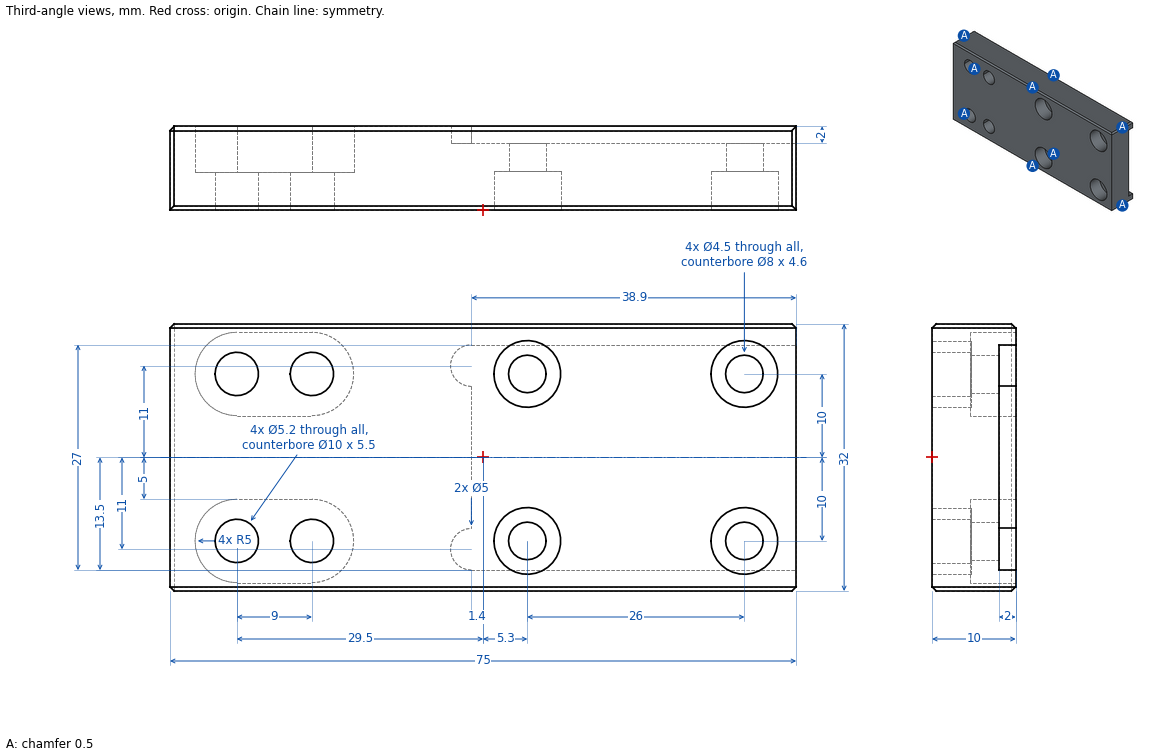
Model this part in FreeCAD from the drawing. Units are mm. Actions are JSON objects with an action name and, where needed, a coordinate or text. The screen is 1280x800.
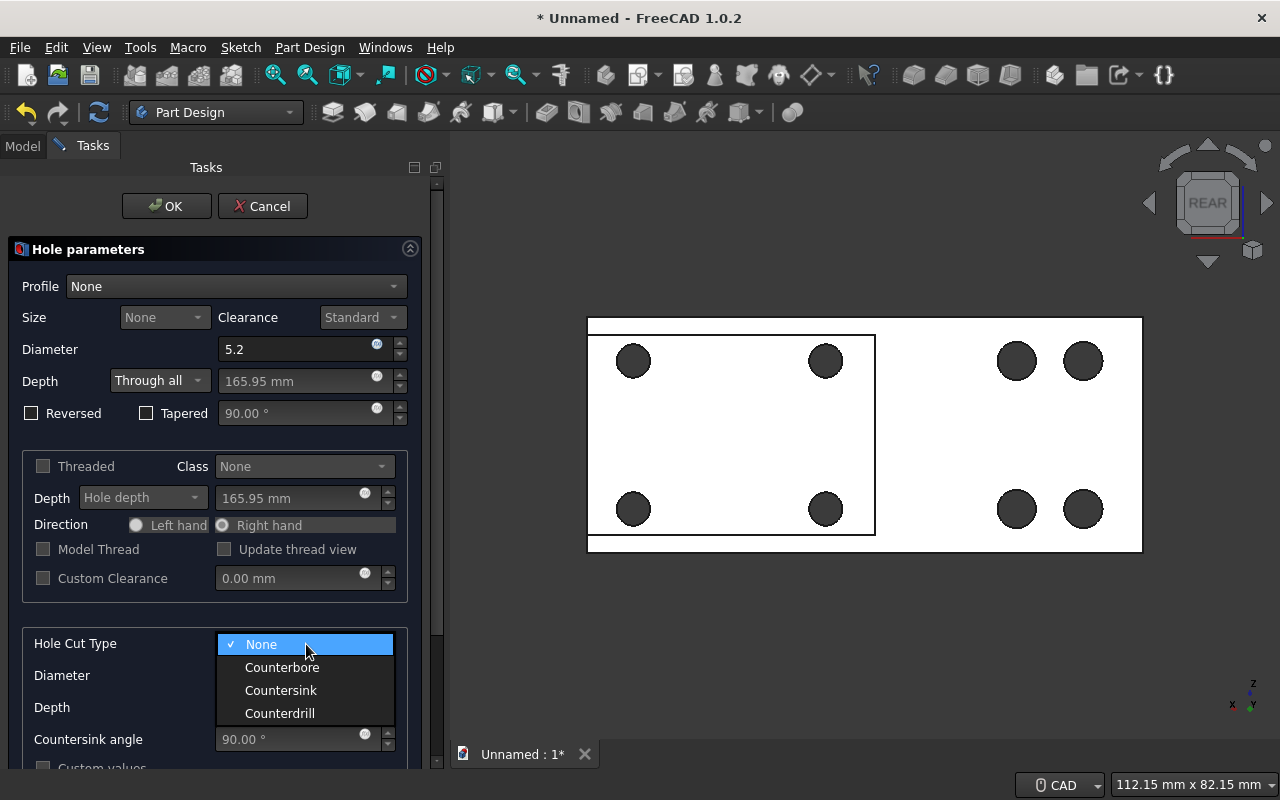
{"action": "left_click", "coordinate": [304, 668]}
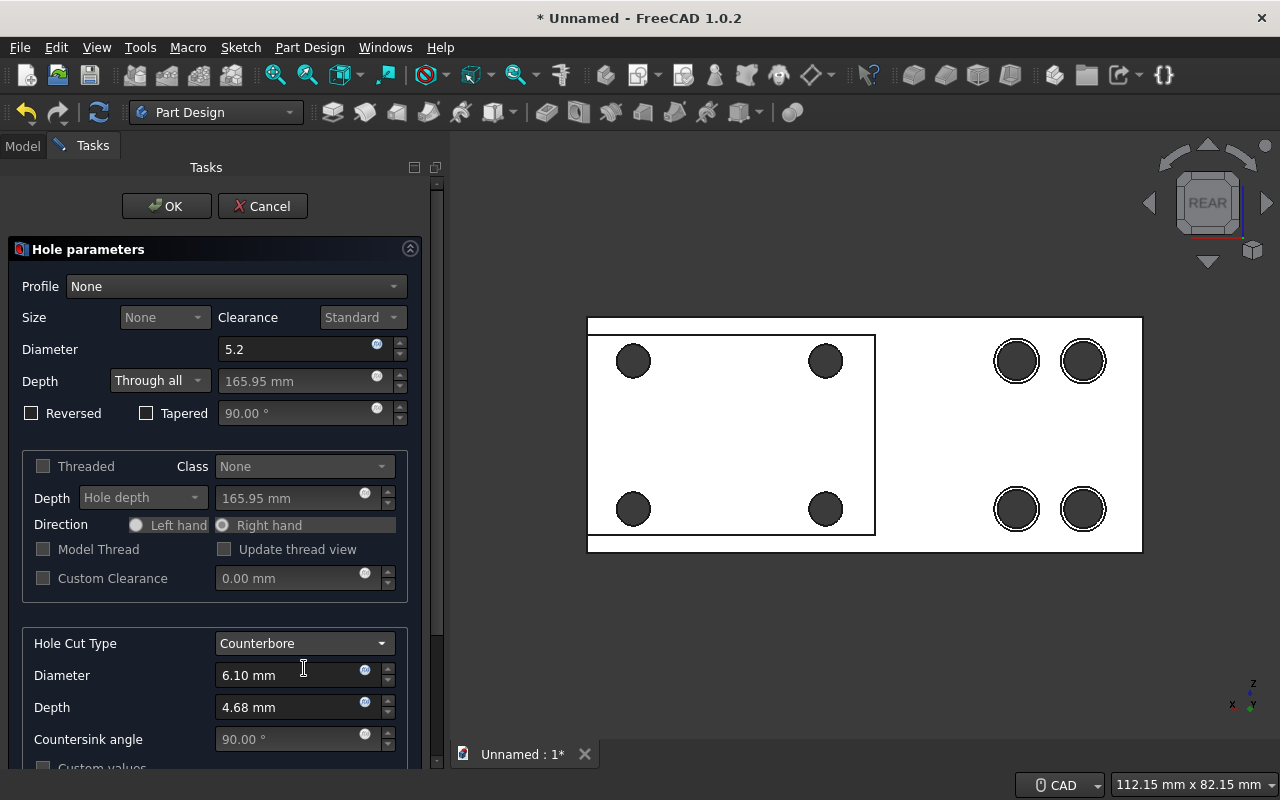
{"action": "triple_click", "coordinate": [298, 675]}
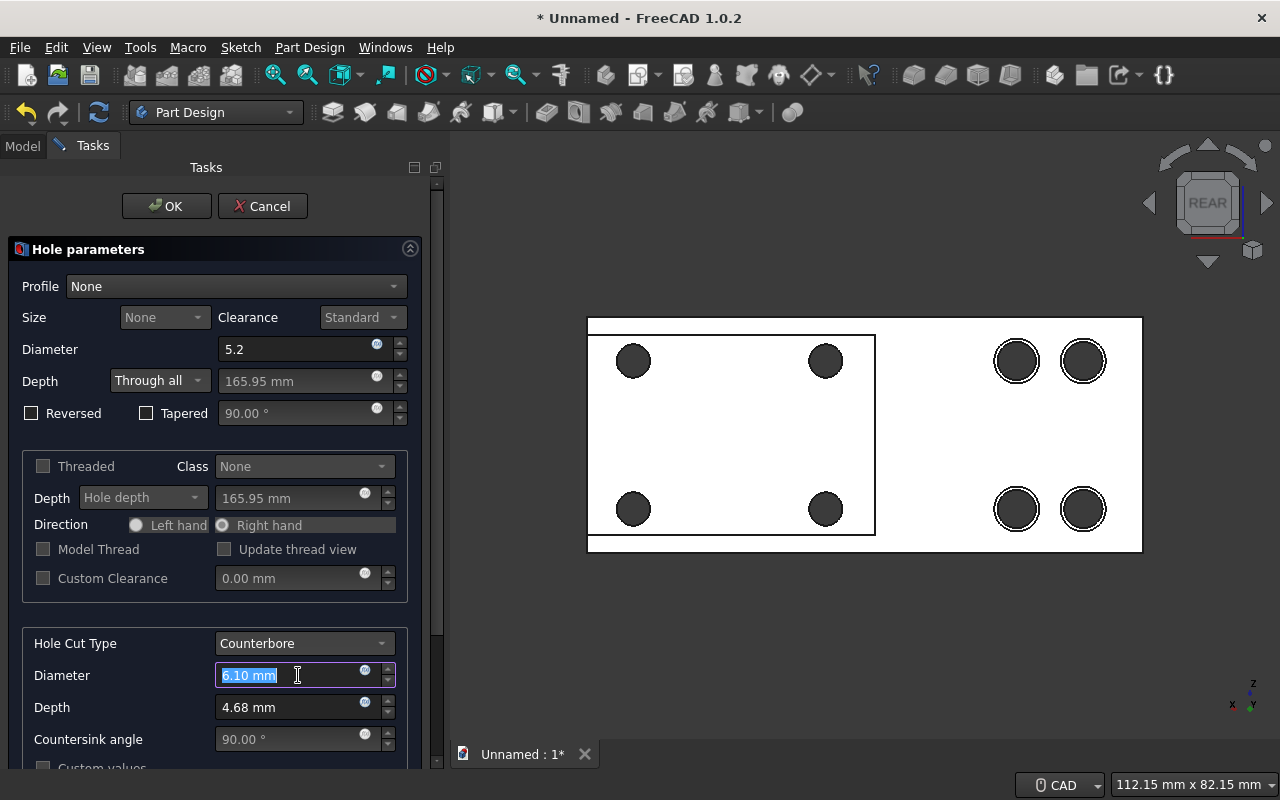
{"action": "type", "text": "10"}
{"action": "key", "text": "Tab"}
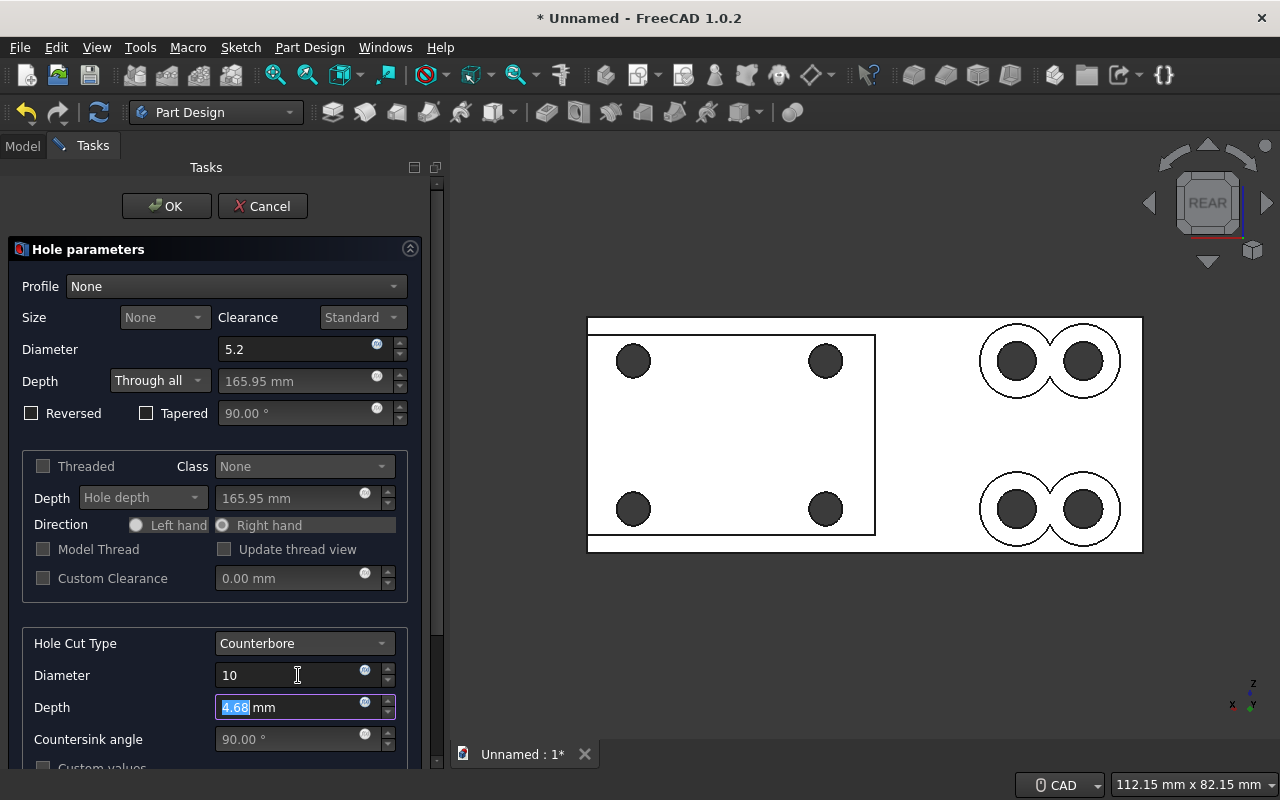
{"action": "type", "text": "5.5"}
{"action": "key", "text": "Tab"}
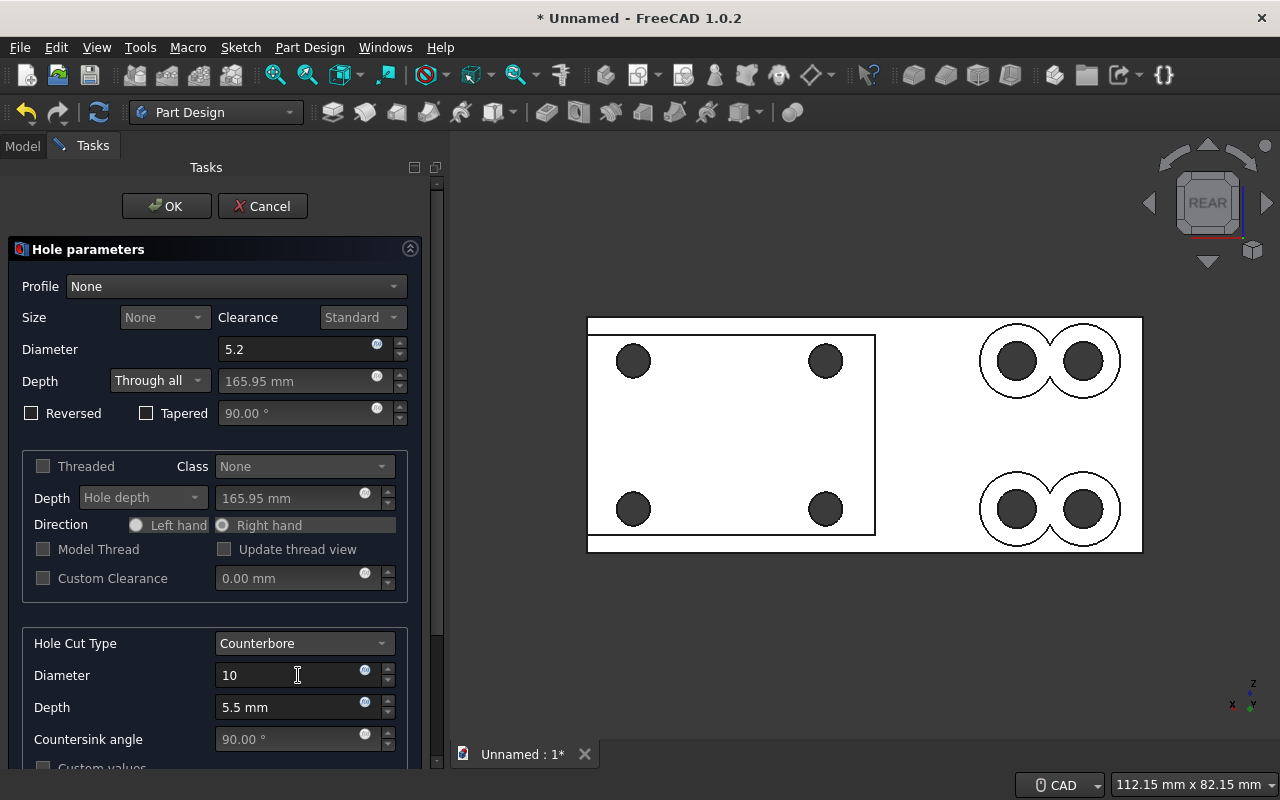
{"action": "left_click", "coordinate": [167, 206]}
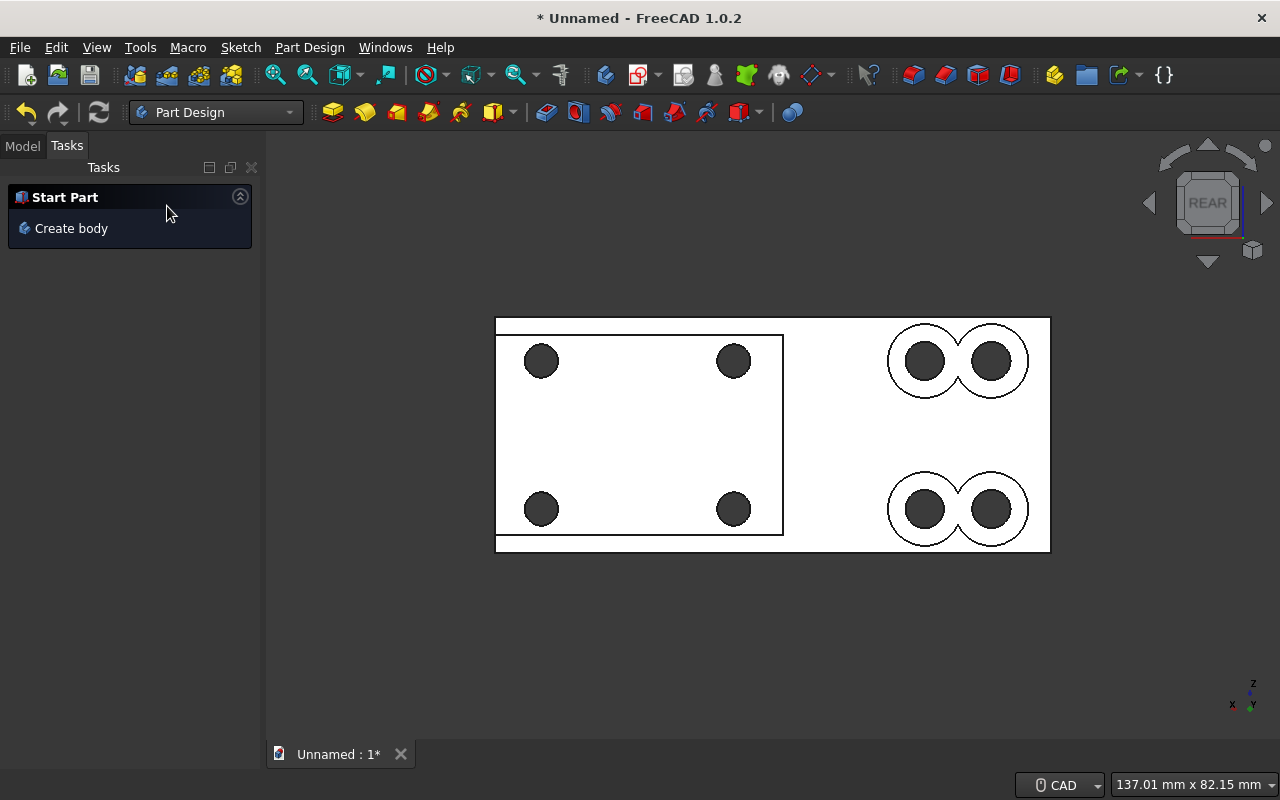
{"action": "left_click", "coordinate": [23, 145]}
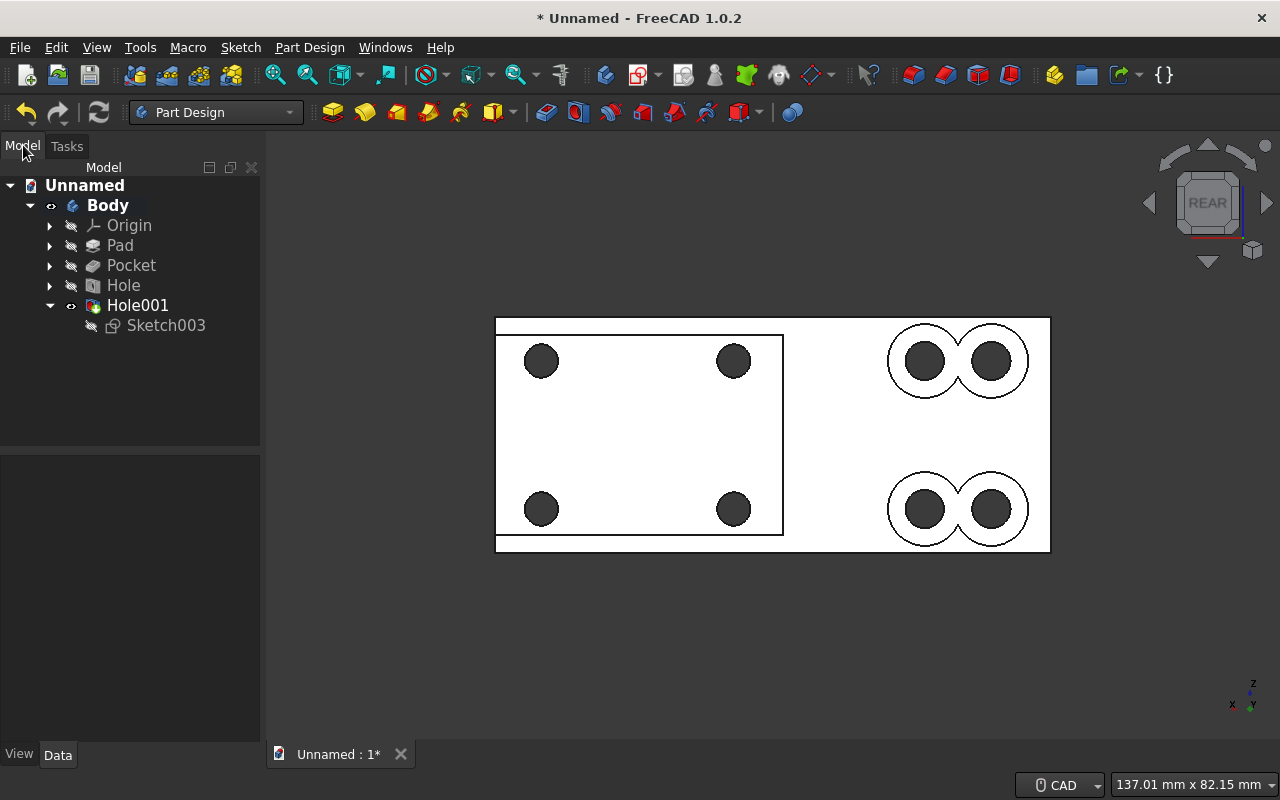
{"action": "left_click", "coordinate": [50, 226]}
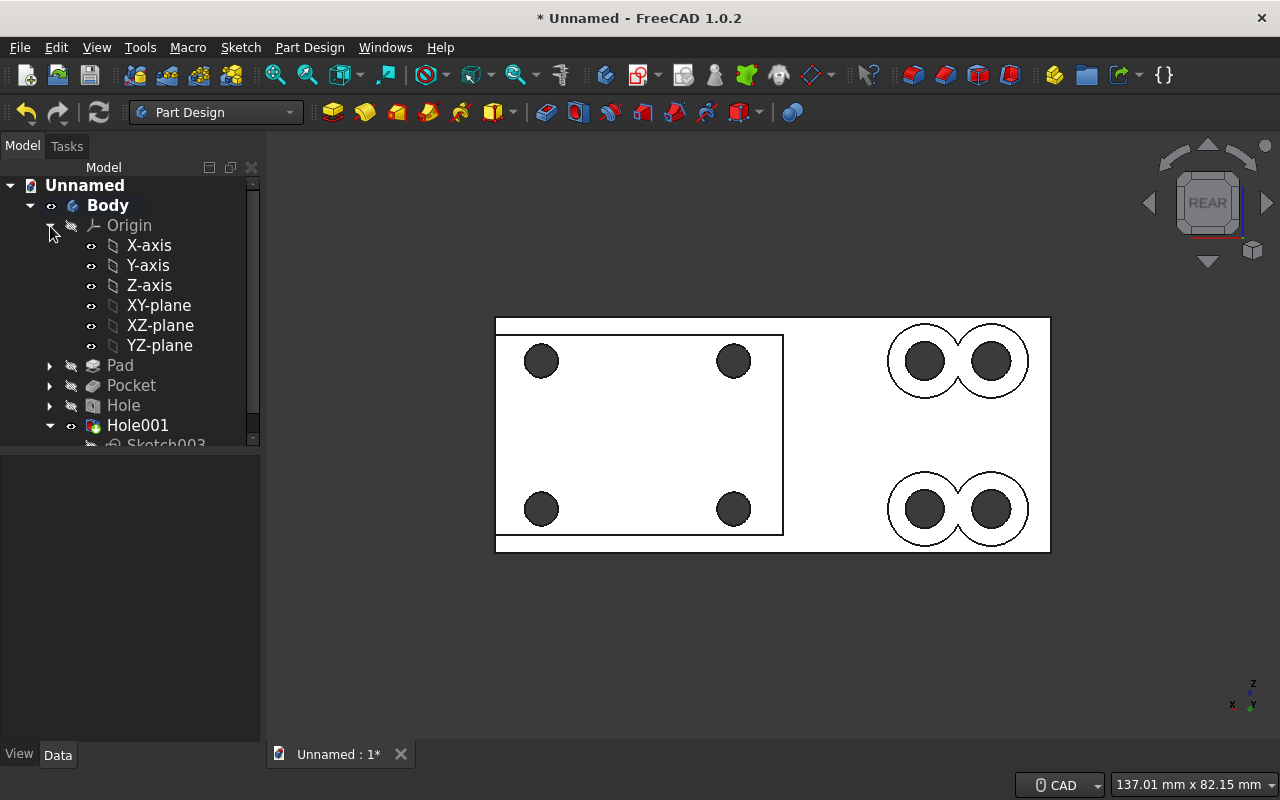
{"action": "left_click", "coordinate": [136, 326]}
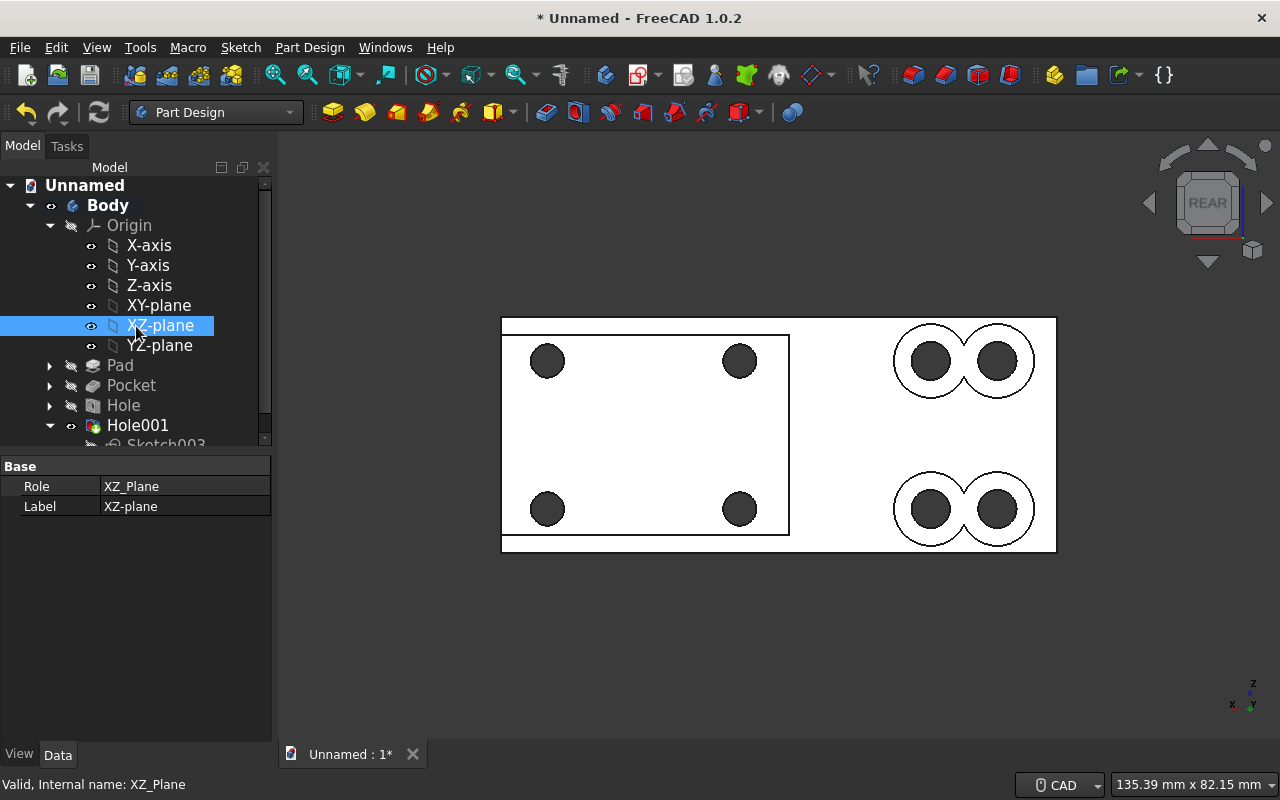
{"action": "left_click", "coordinate": [812, 76]}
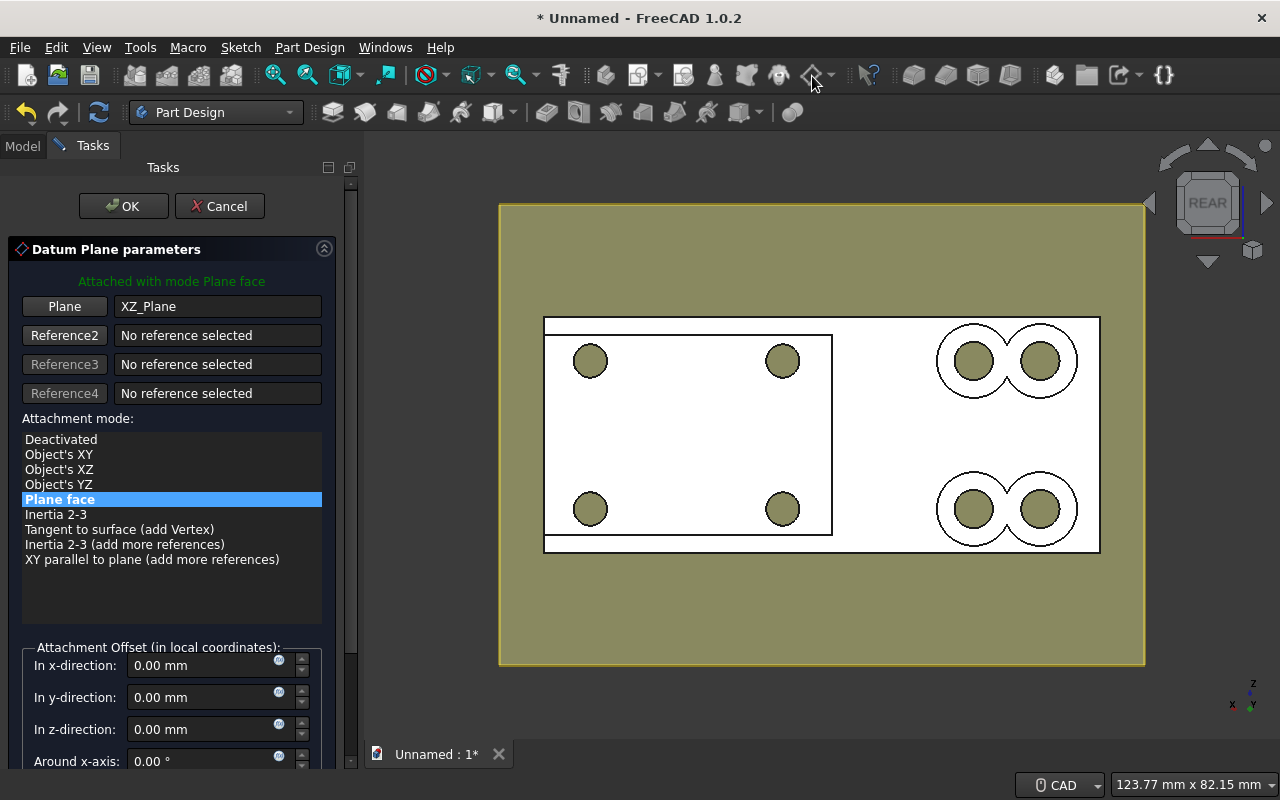
{"action": "triple_click", "coordinate": [210, 729]}